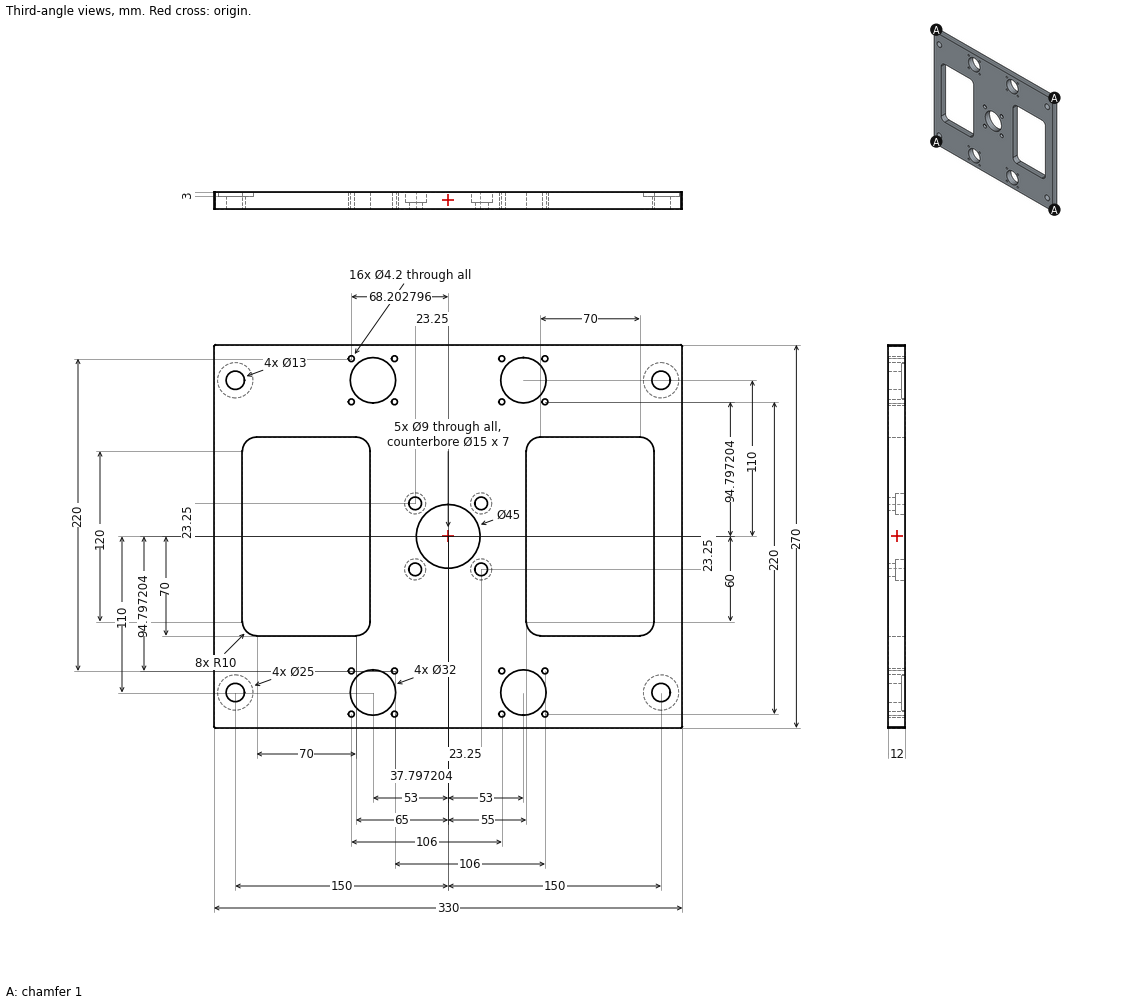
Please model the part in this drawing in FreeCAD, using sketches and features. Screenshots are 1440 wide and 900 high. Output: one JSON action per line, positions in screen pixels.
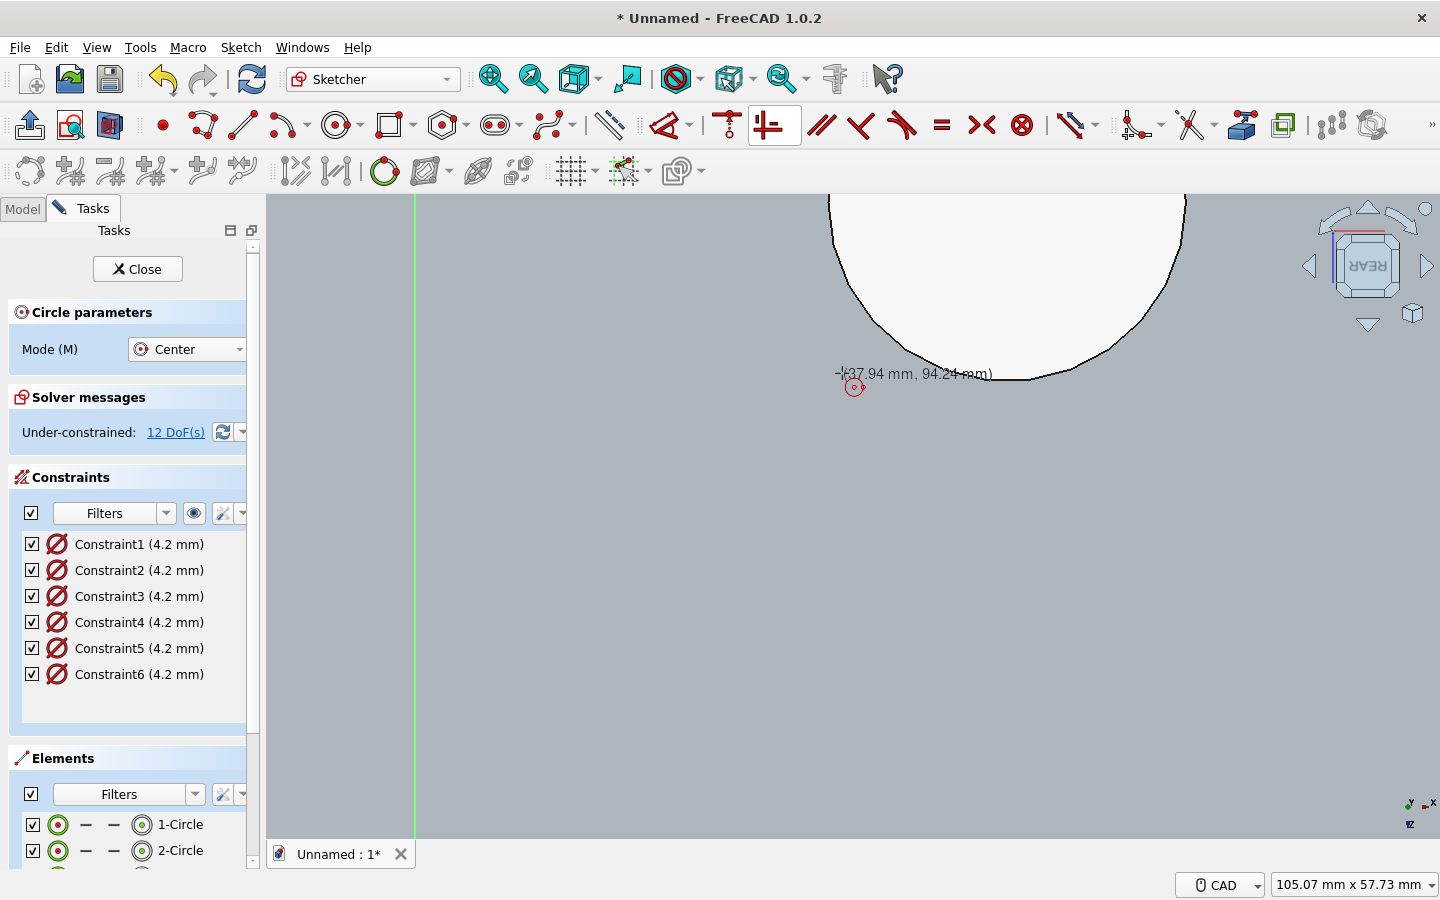
{"action": "scroll", "coordinate": [842, 373], "scroll_direction": "down", "scroll_amount": 10}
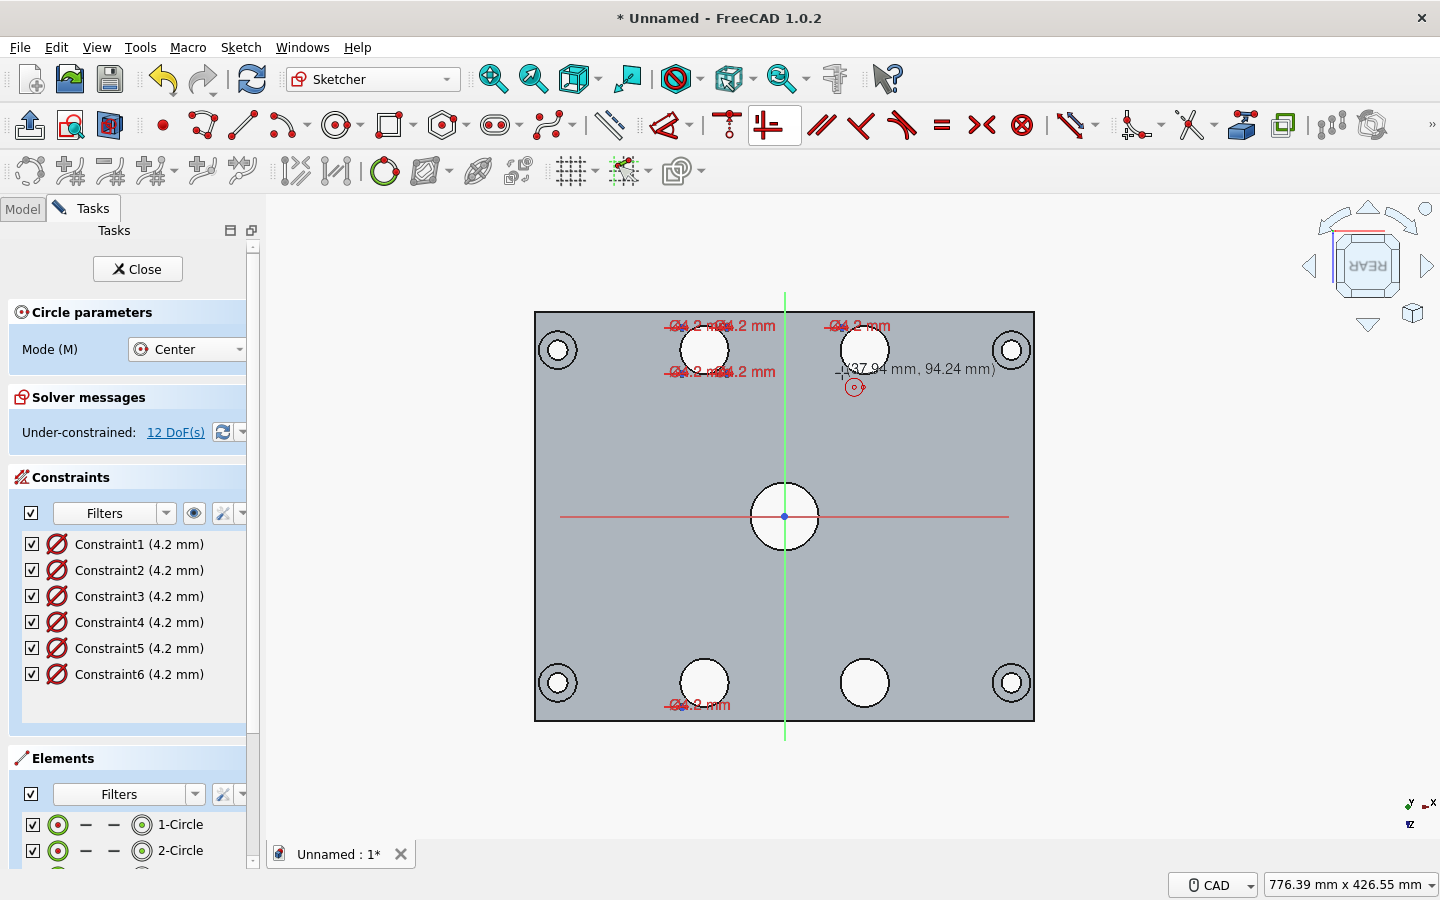
{"action": "left_click", "coordinate": [842, 373]}
{"action": "mouse_move", "coordinate": [844, 371]}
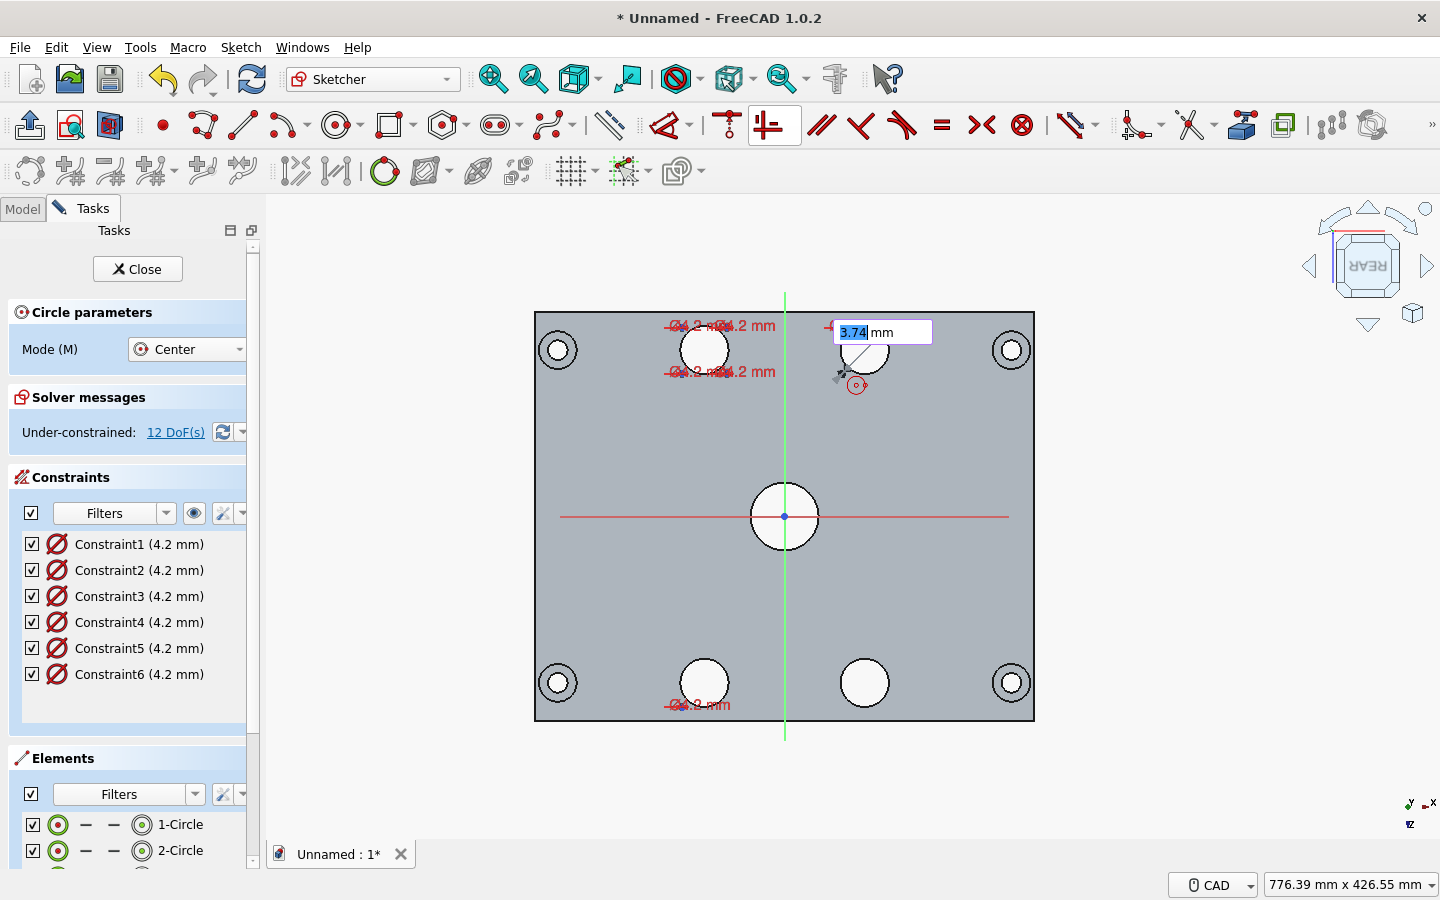
{"action": "type", "text": "4.2"}
{"action": "key", "text": "Return"}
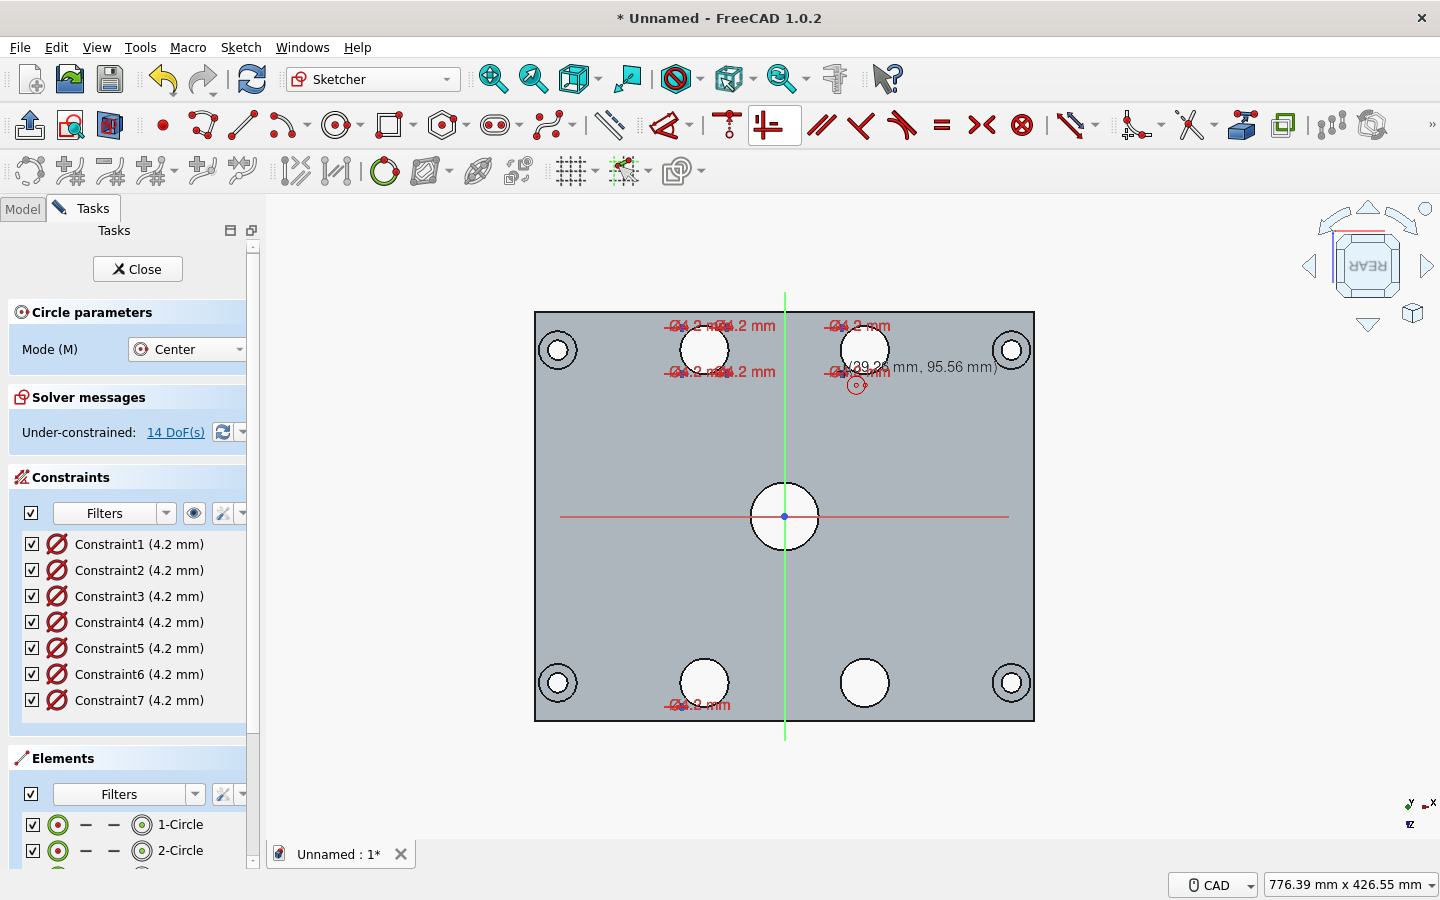
{"action": "scroll", "coordinate": [888, 373], "scroll_direction": "up", "scroll_amount": 10}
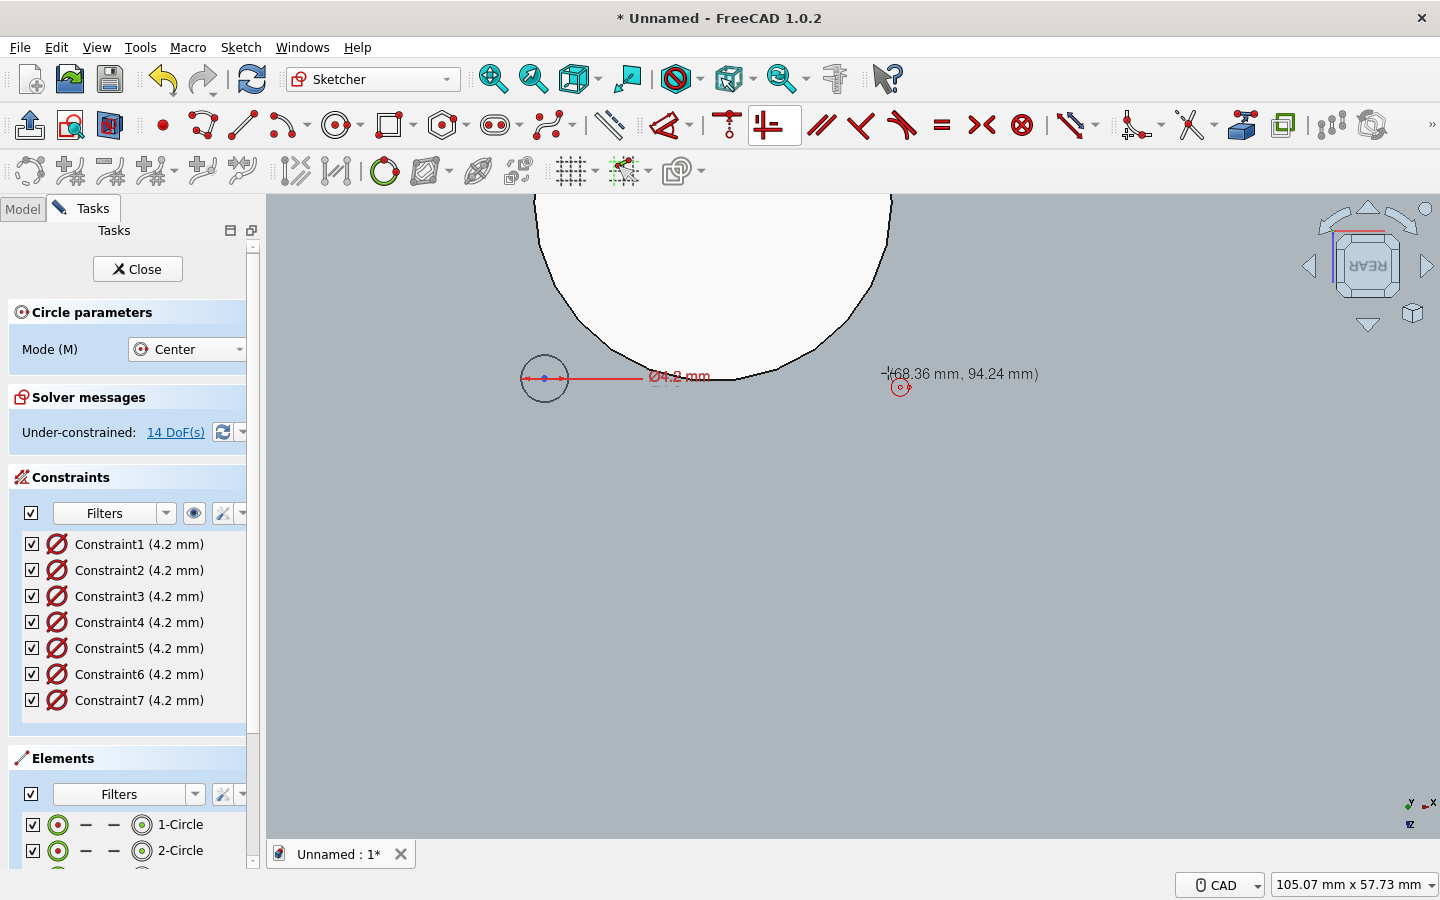
{"action": "scroll", "coordinate": [888, 373], "scroll_direction": "down", "scroll_amount": 10}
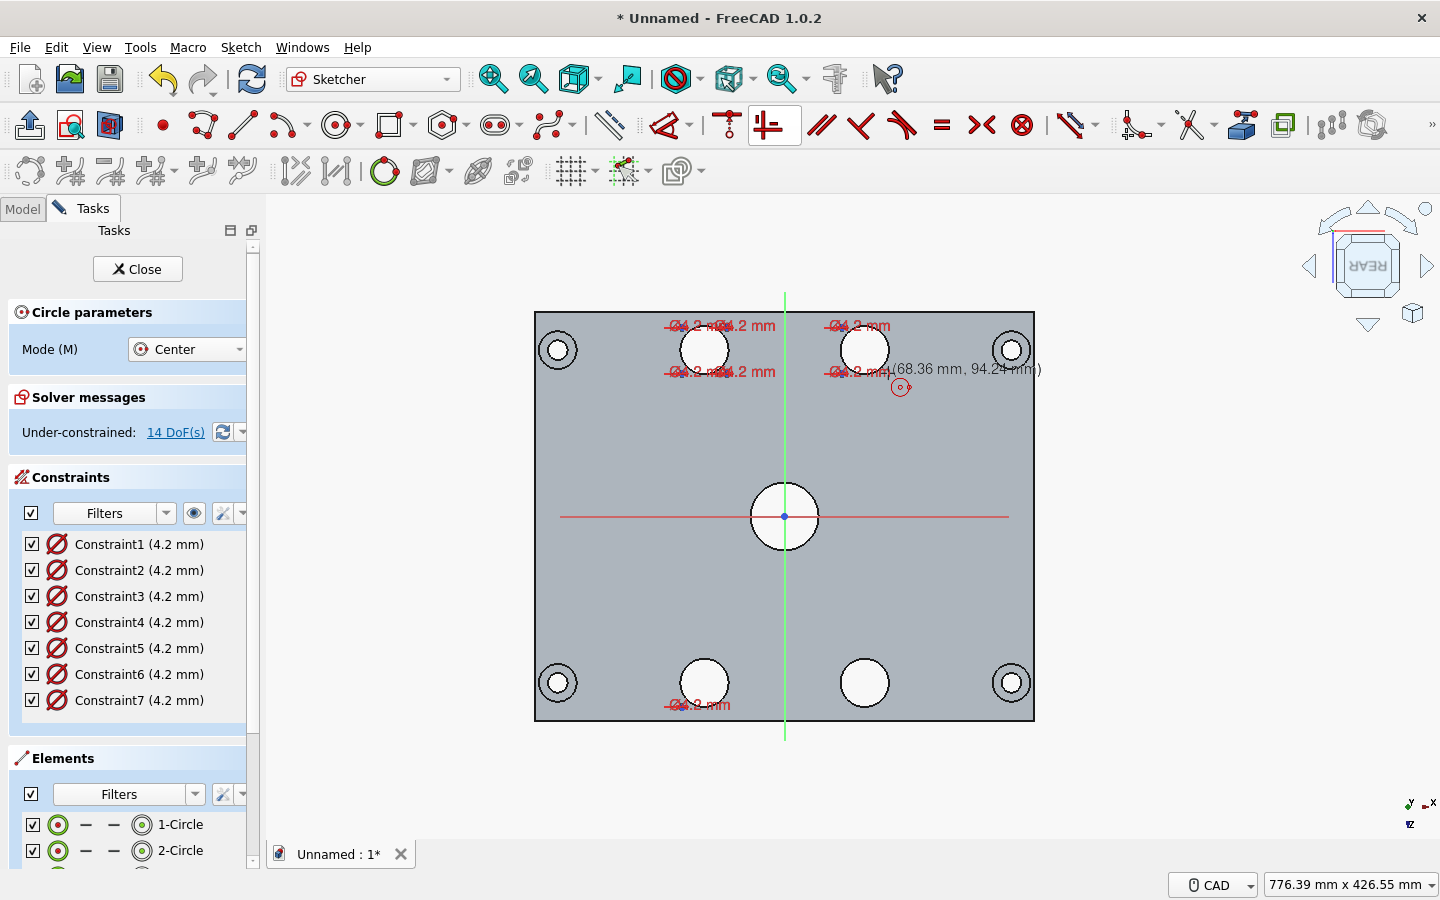
{"action": "left_click", "coordinate": [888, 373]}
{"action": "mouse_move", "coordinate": [890, 371]}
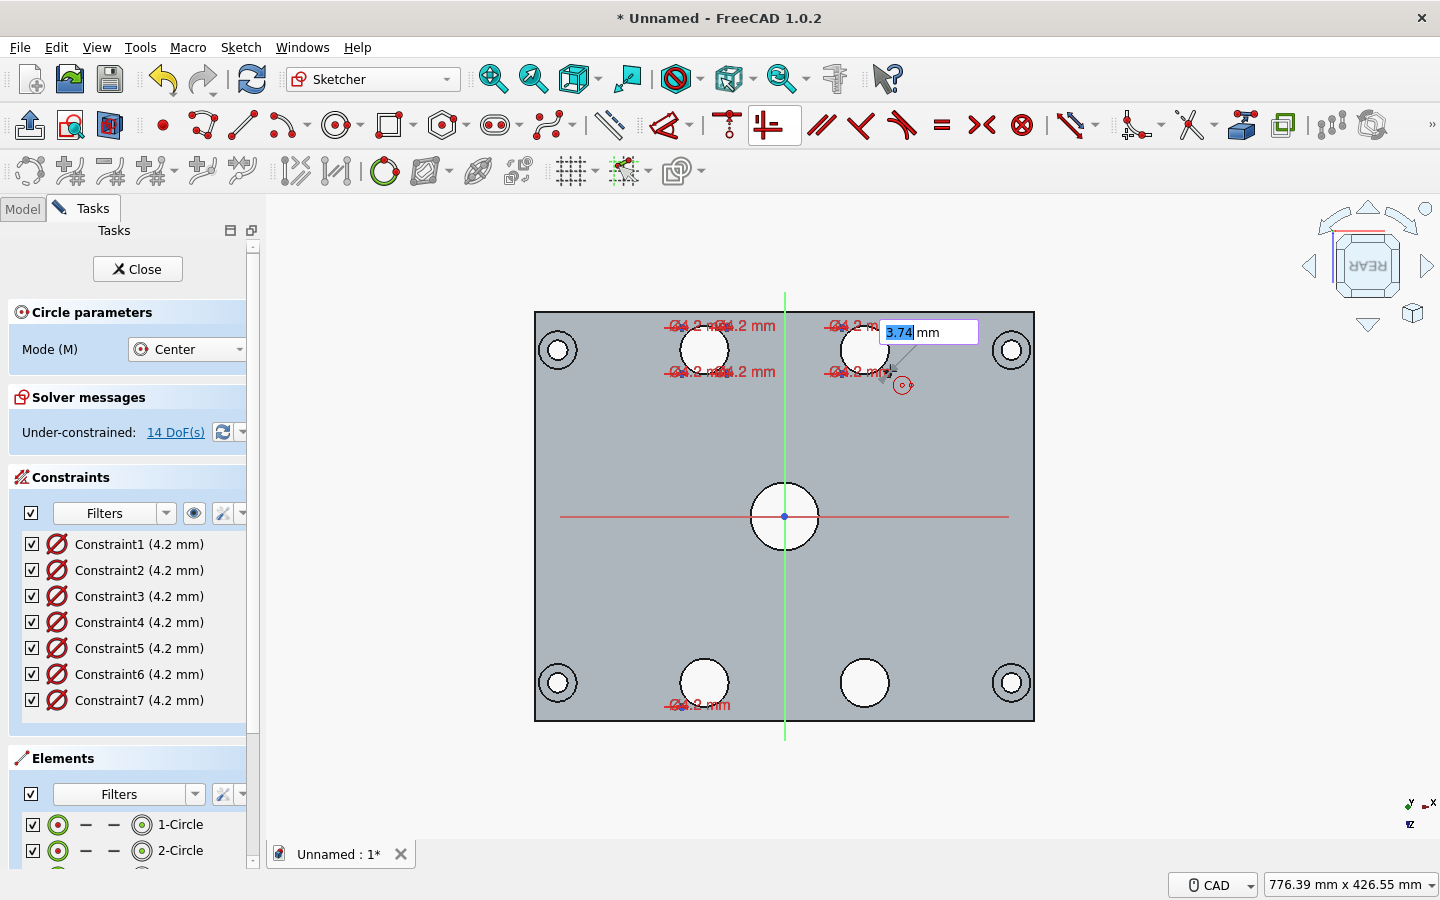
{"action": "type", "text": "4.2"}
{"action": "key", "text": "Return"}